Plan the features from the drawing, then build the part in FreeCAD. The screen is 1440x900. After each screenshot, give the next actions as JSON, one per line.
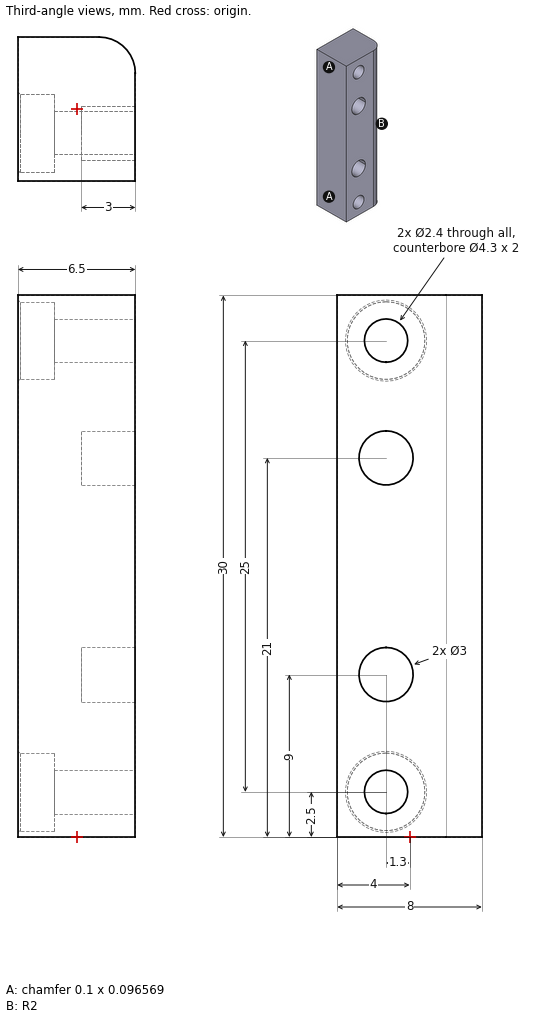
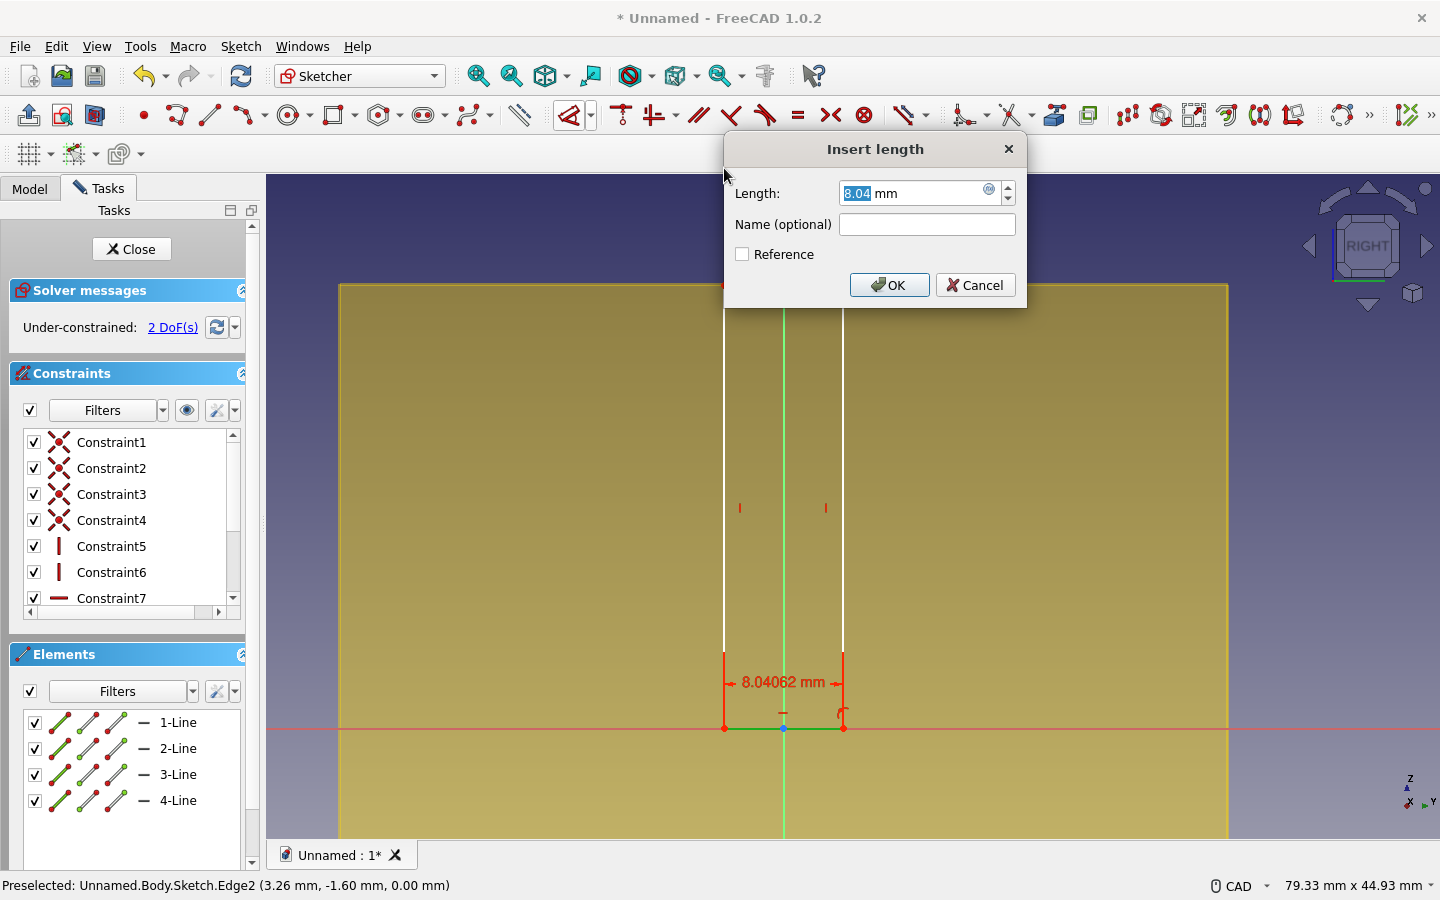
{"action": "type", "text": "8"}
{"action": "key", "text": "Return"}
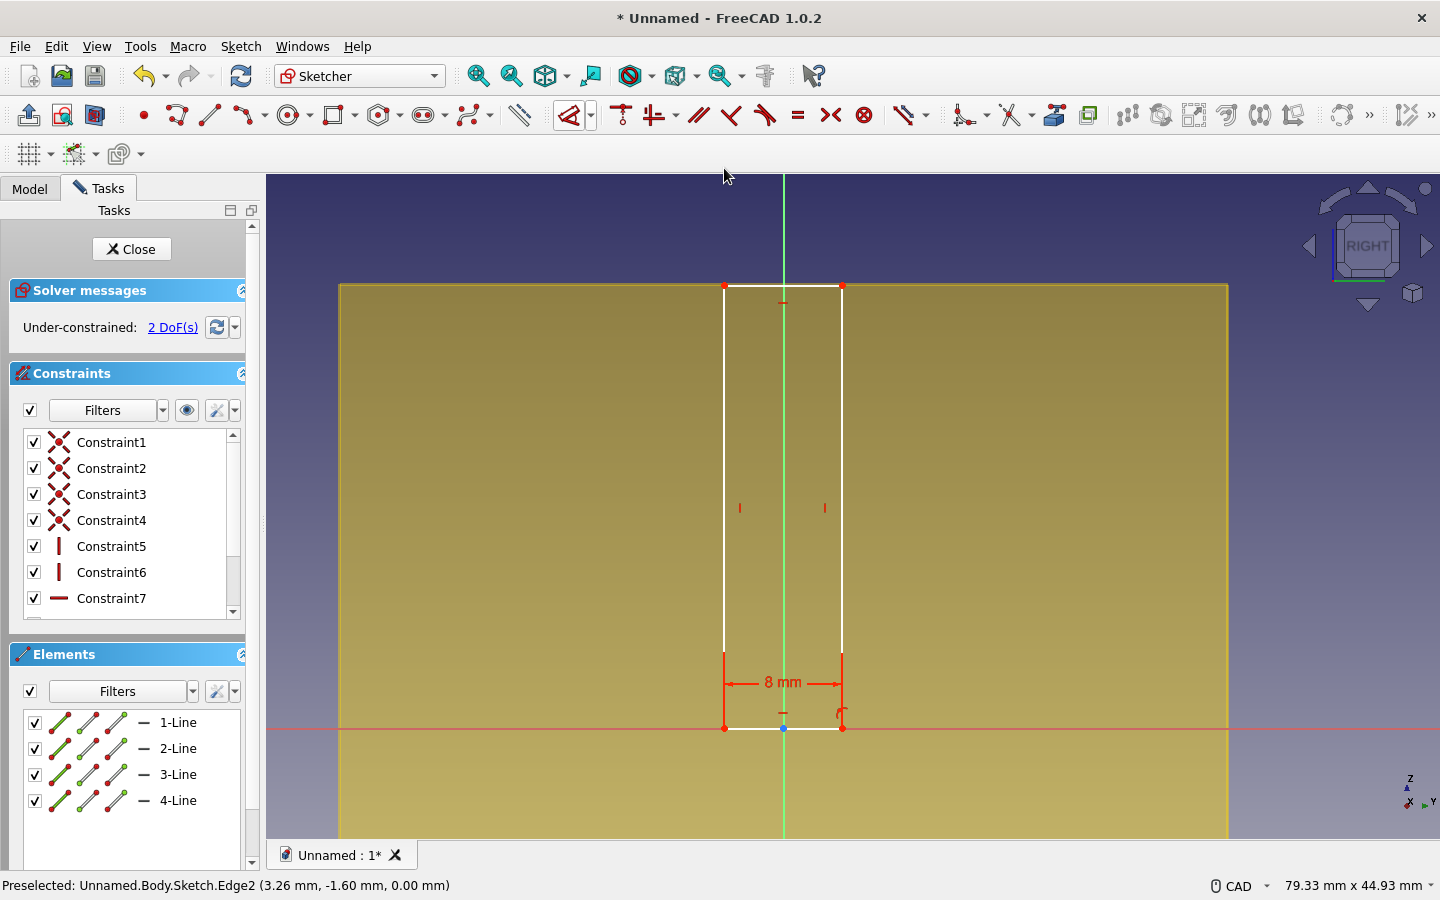
{"action": "left_click", "coordinate": [724, 419]}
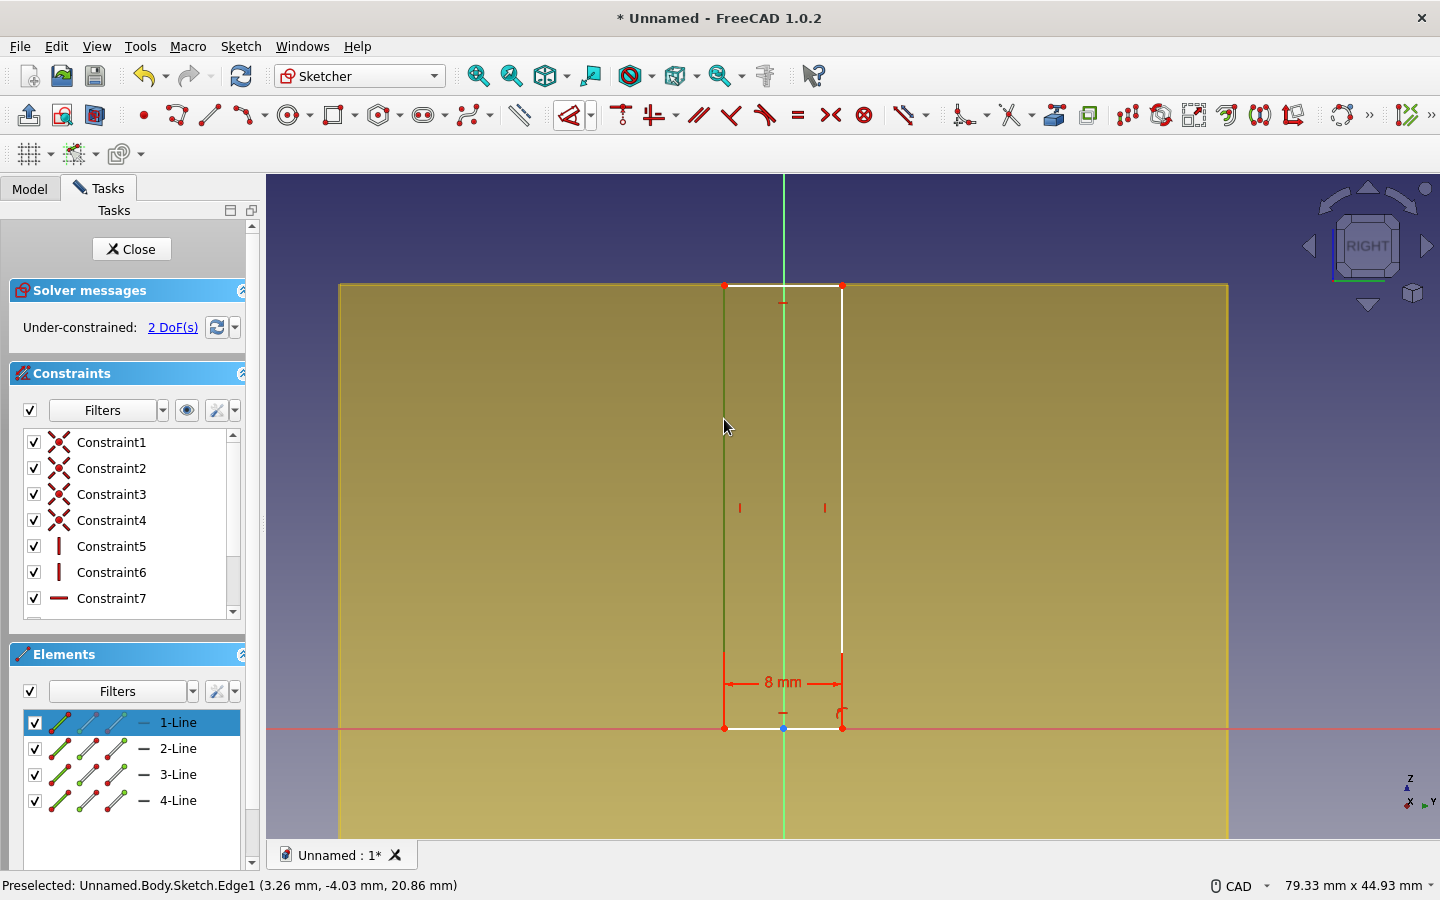
{"action": "left_click", "coordinate": [590, 116]}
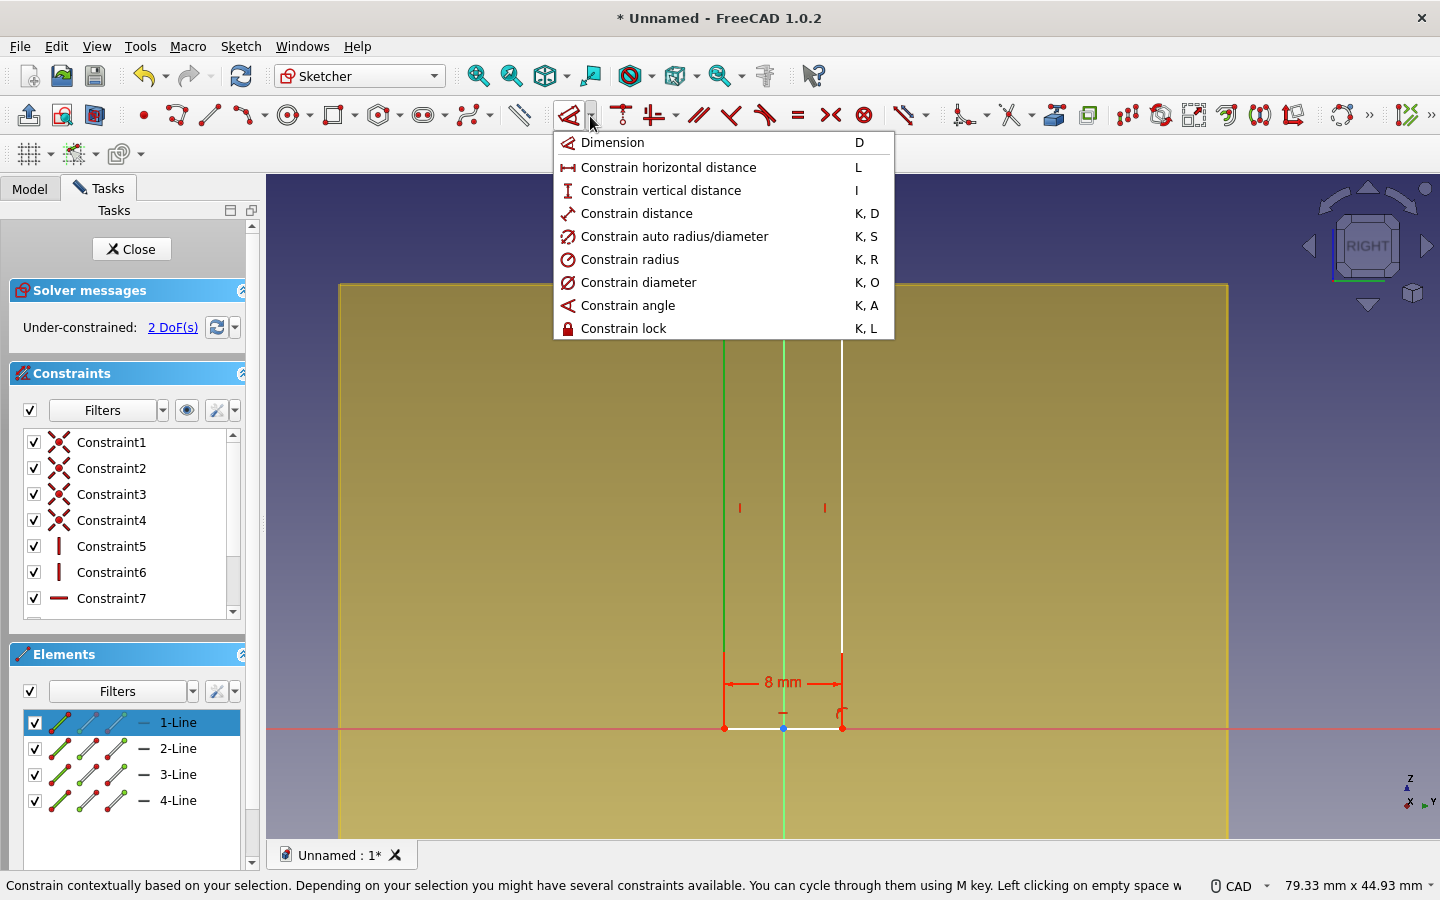
{"action": "left_click", "coordinate": [724, 190]}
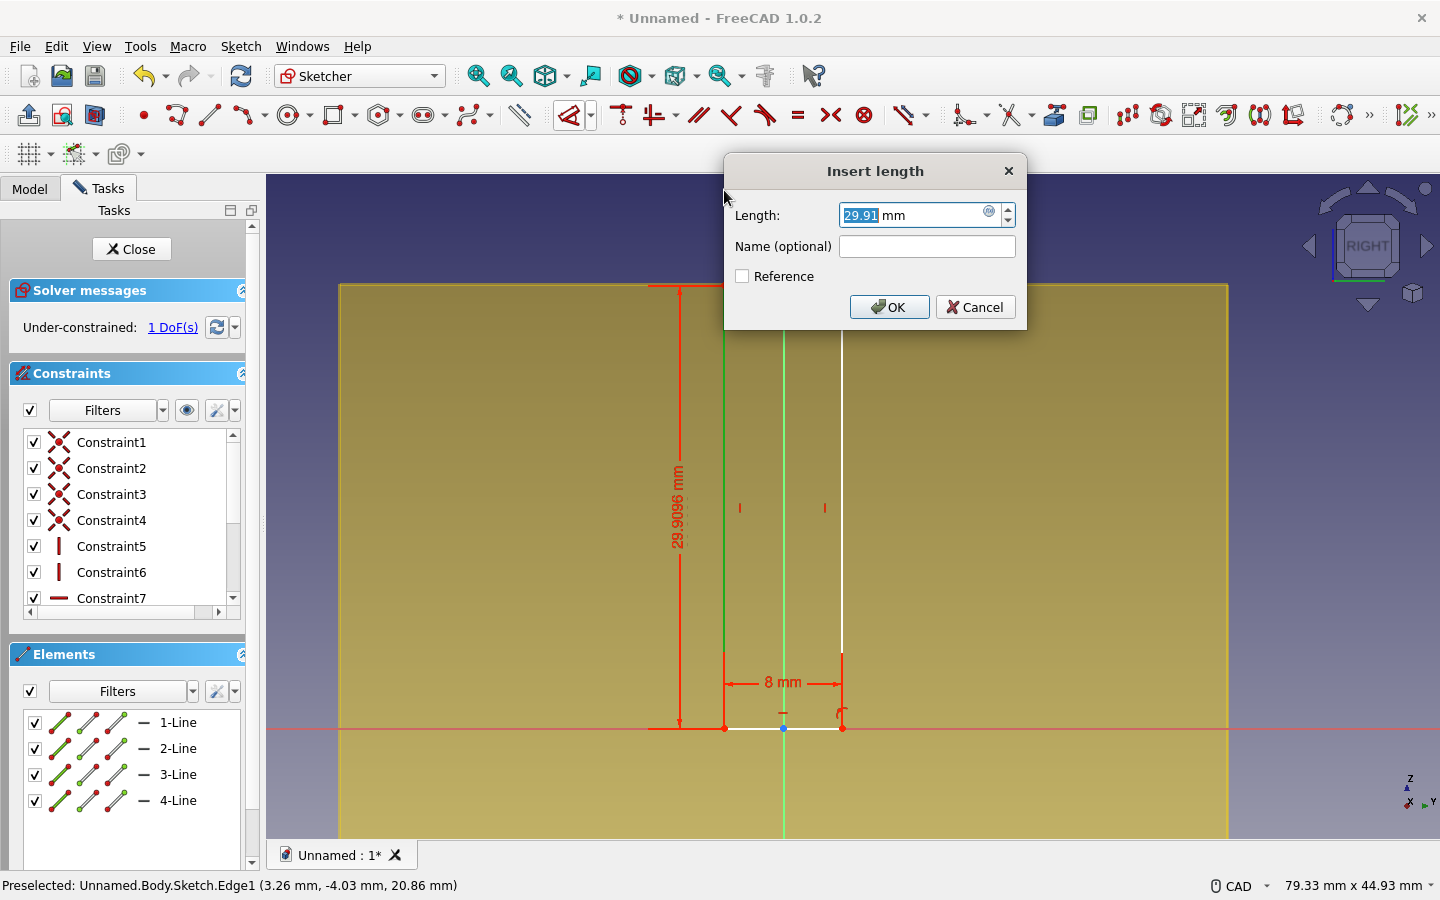
{"action": "type", "text": "30"}
{"action": "key", "text": "Return"}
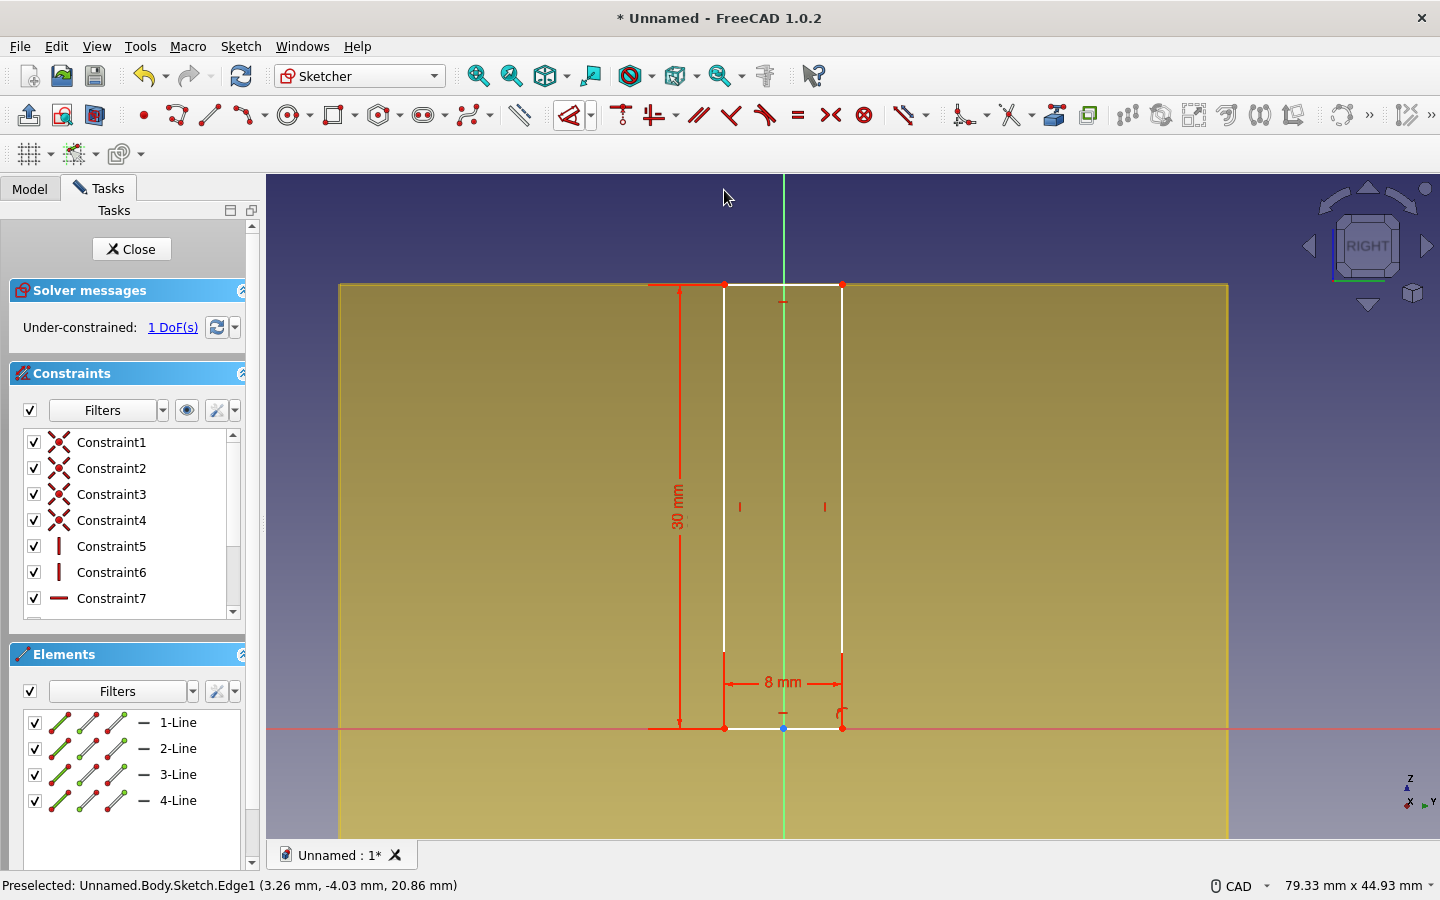
{"action": "left_click", "coordinate": [724, 285]}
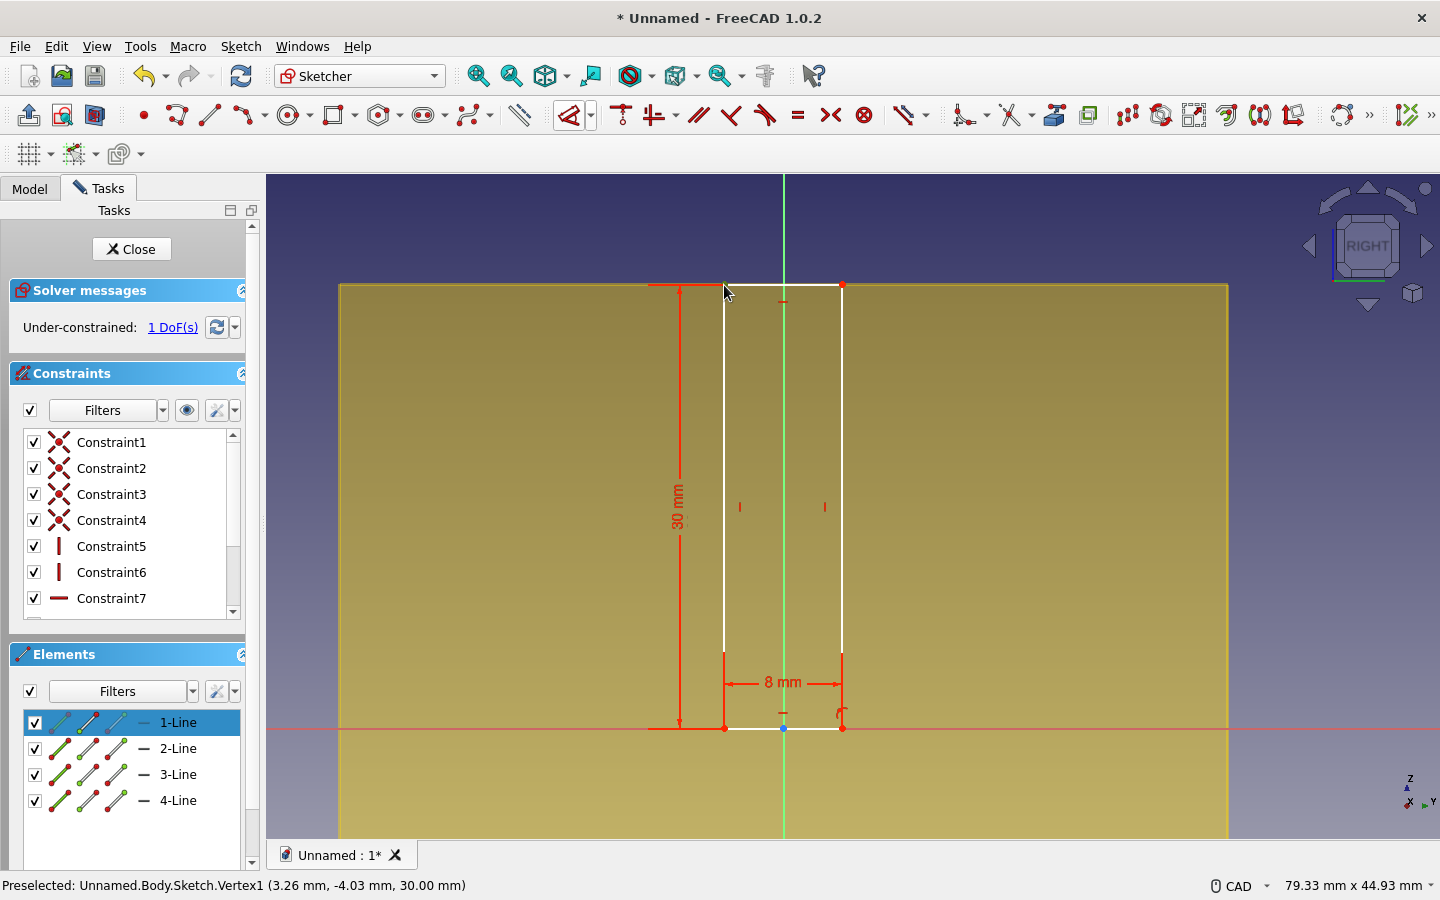
{"action": "left_click", "coordinate": [590, 116]}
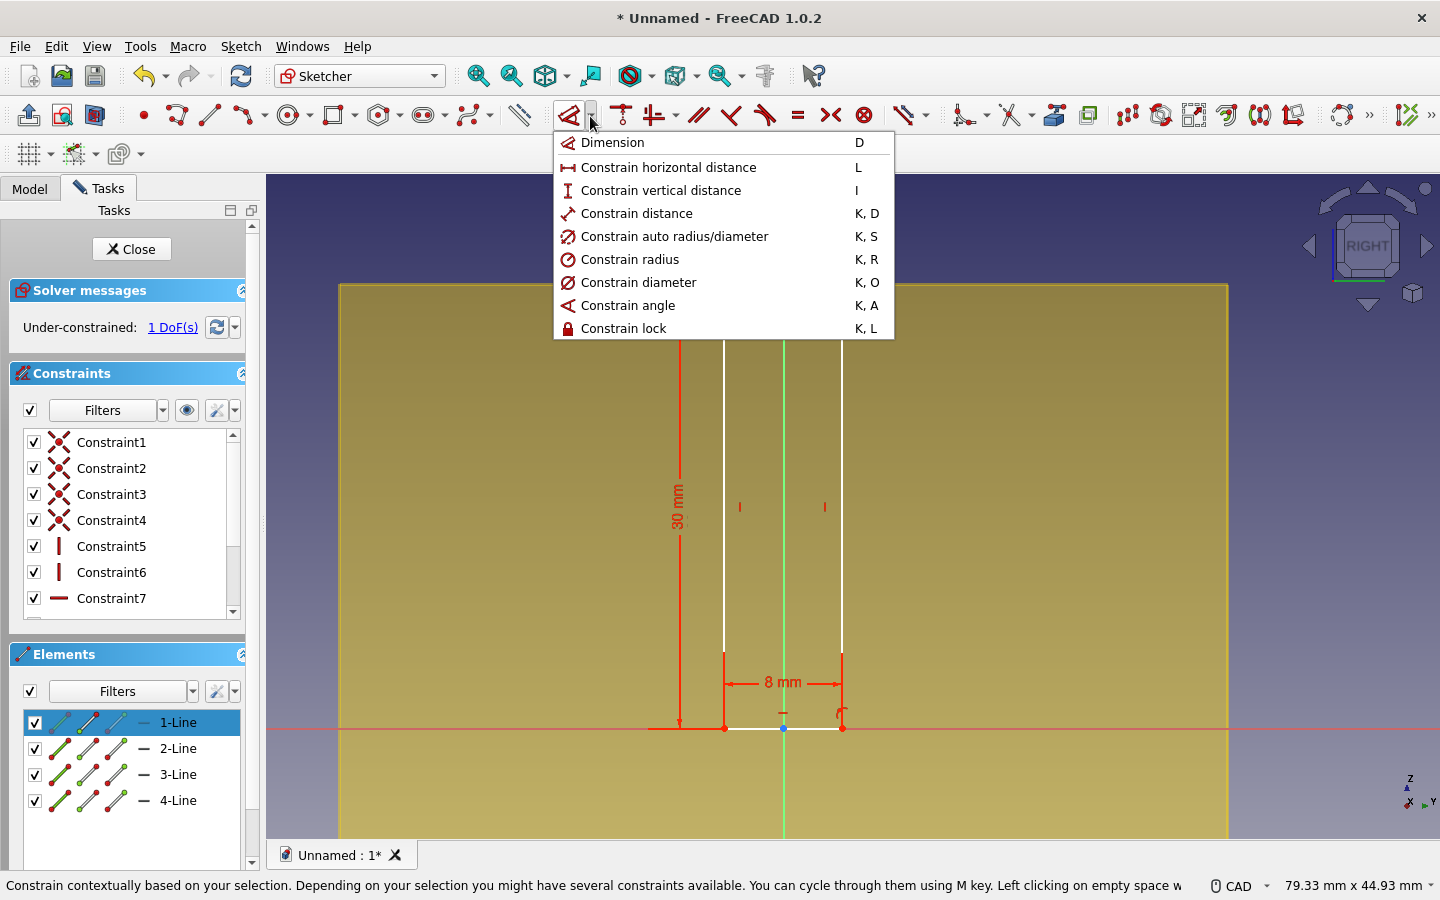
{"action": "left_click", "coordinate": [724, 168]}